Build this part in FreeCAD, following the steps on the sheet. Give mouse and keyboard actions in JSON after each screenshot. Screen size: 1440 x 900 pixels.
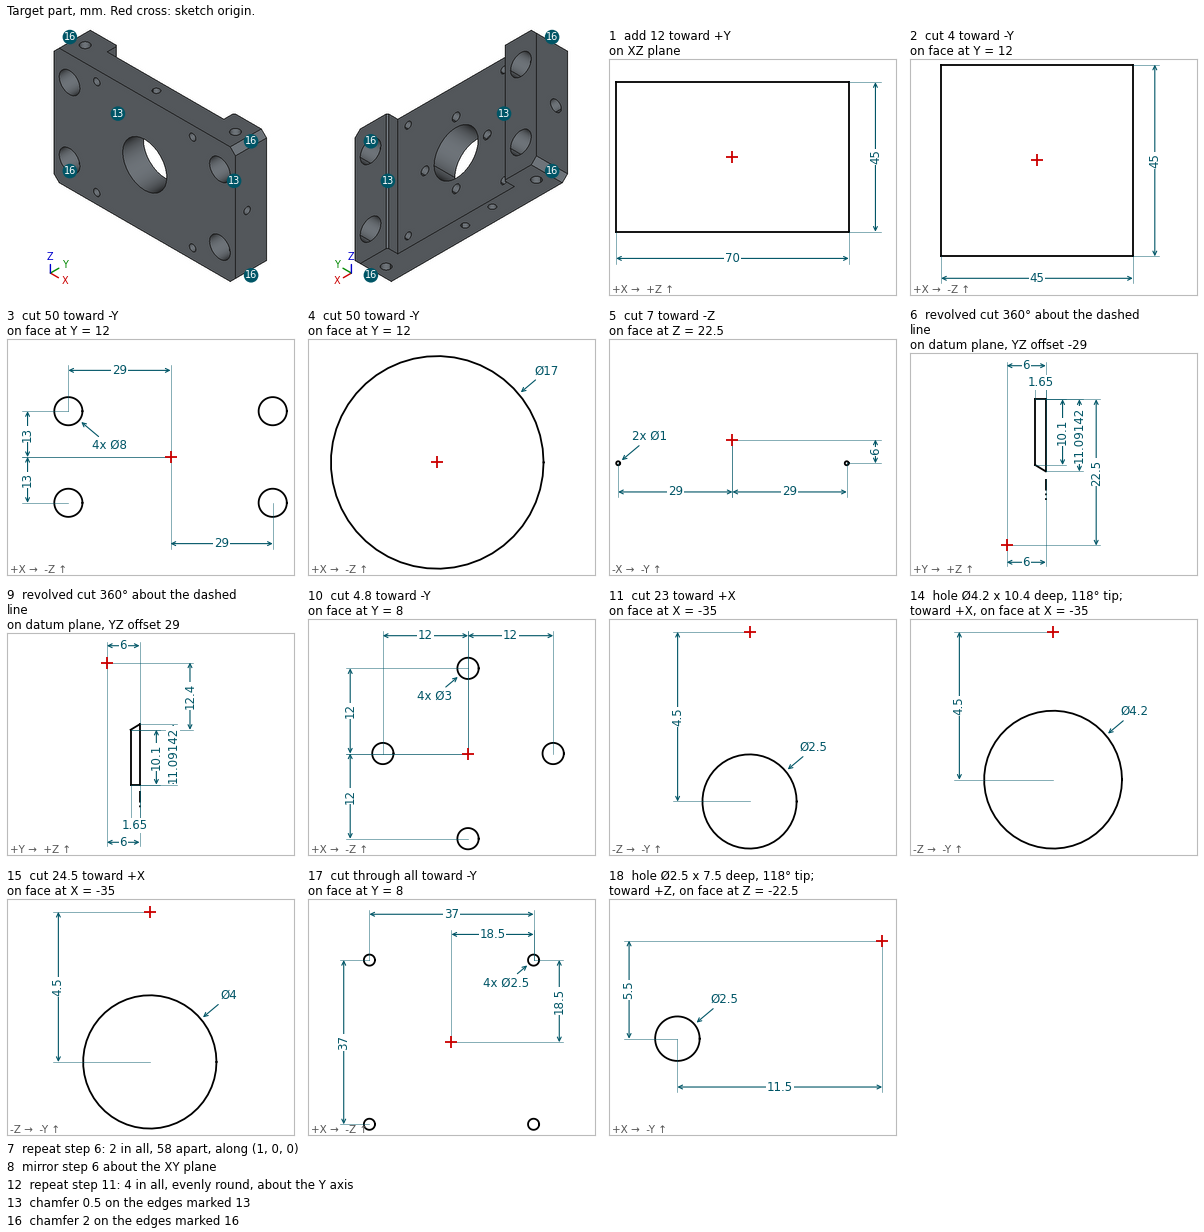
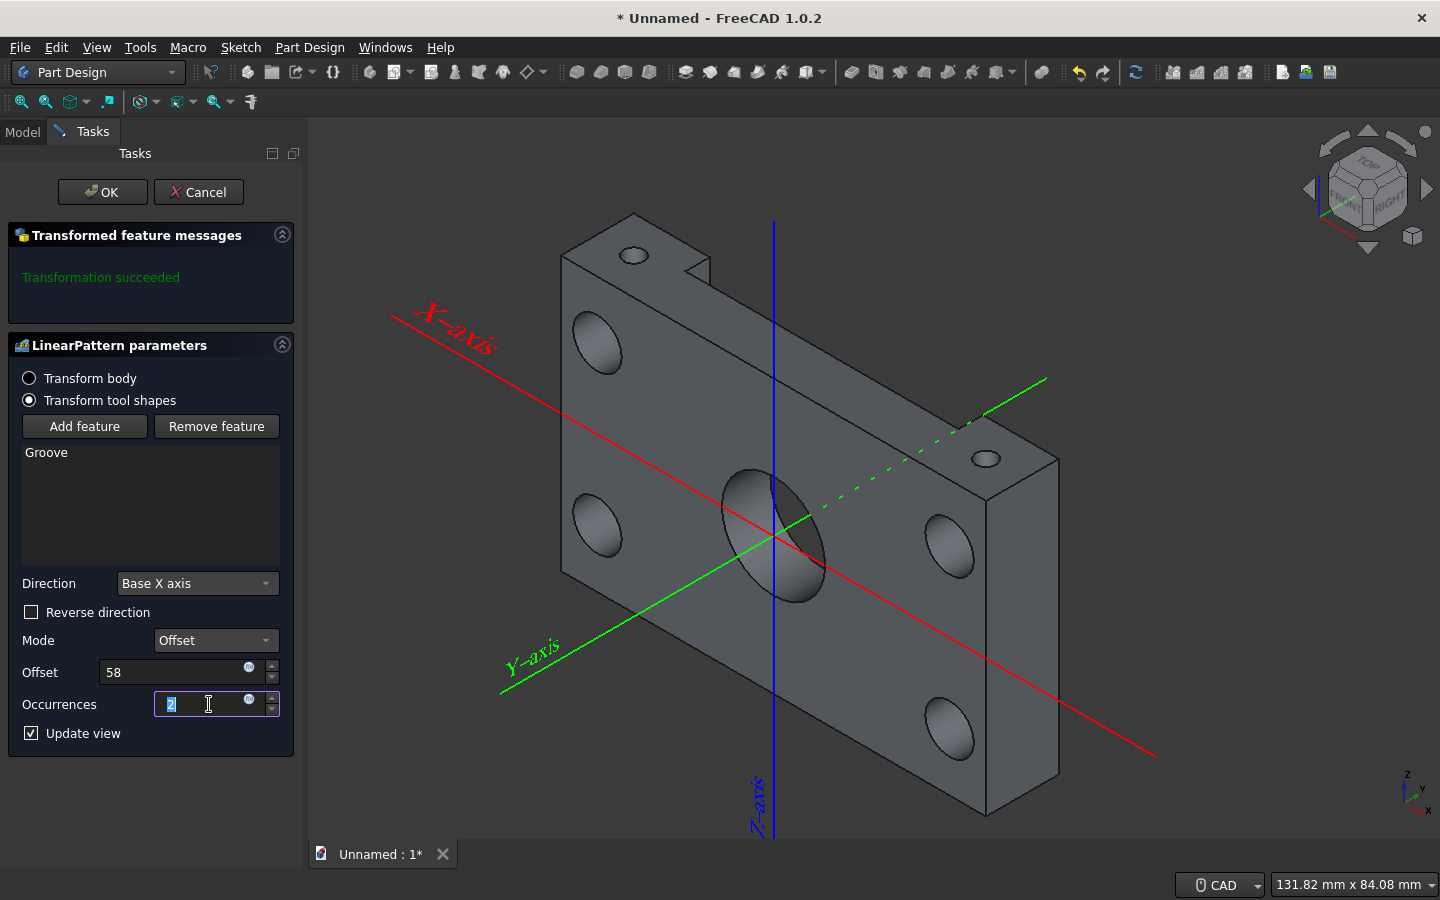
{"action": "type", "text": "2"}
{"action": "key", "text": "Tab"}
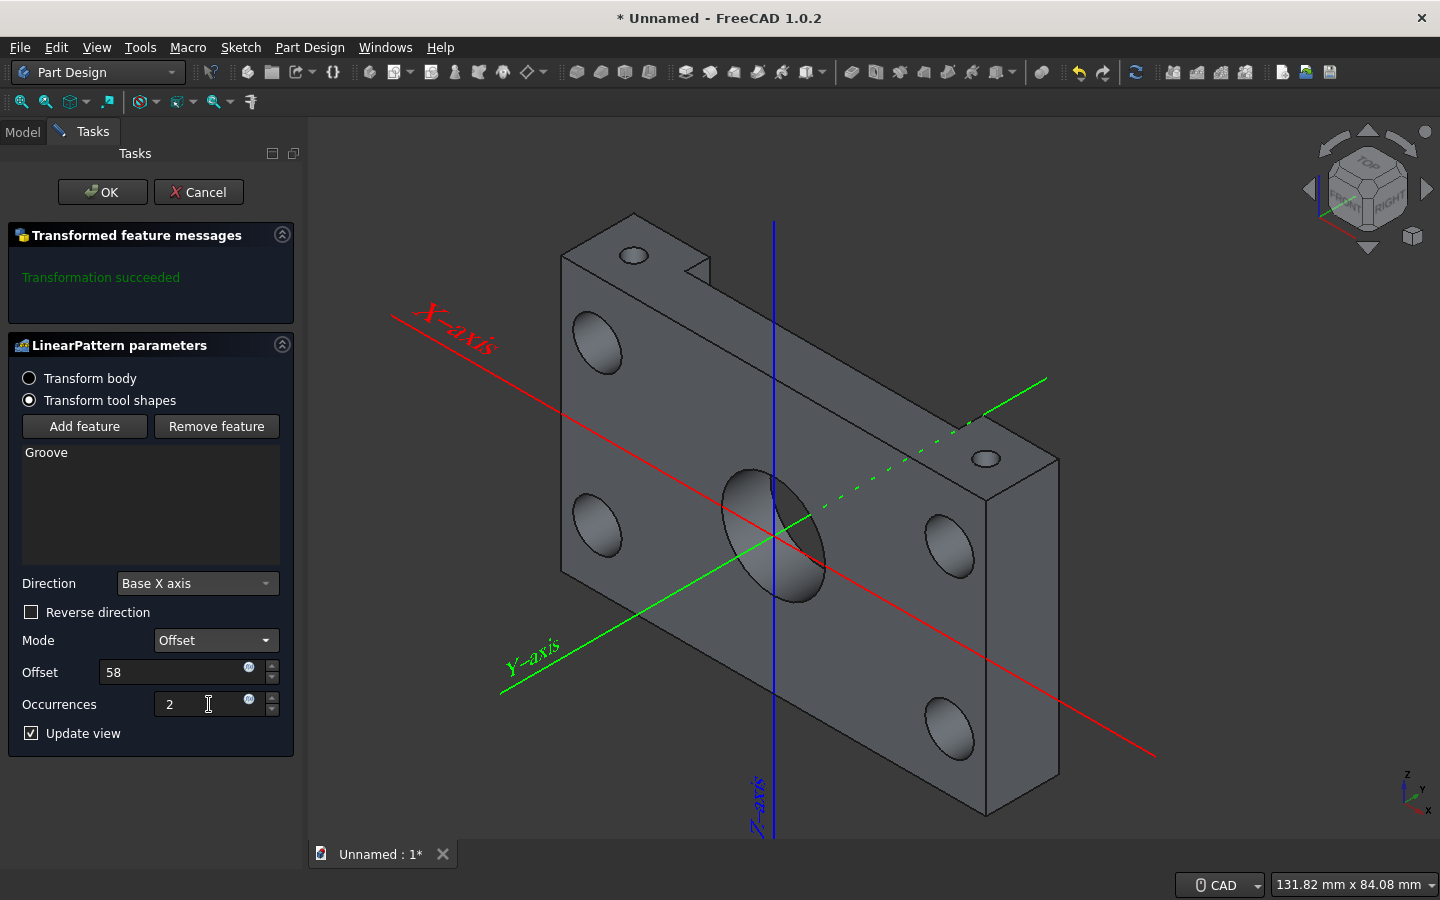
{"action": "left_click", "coordinate": [103, 192]}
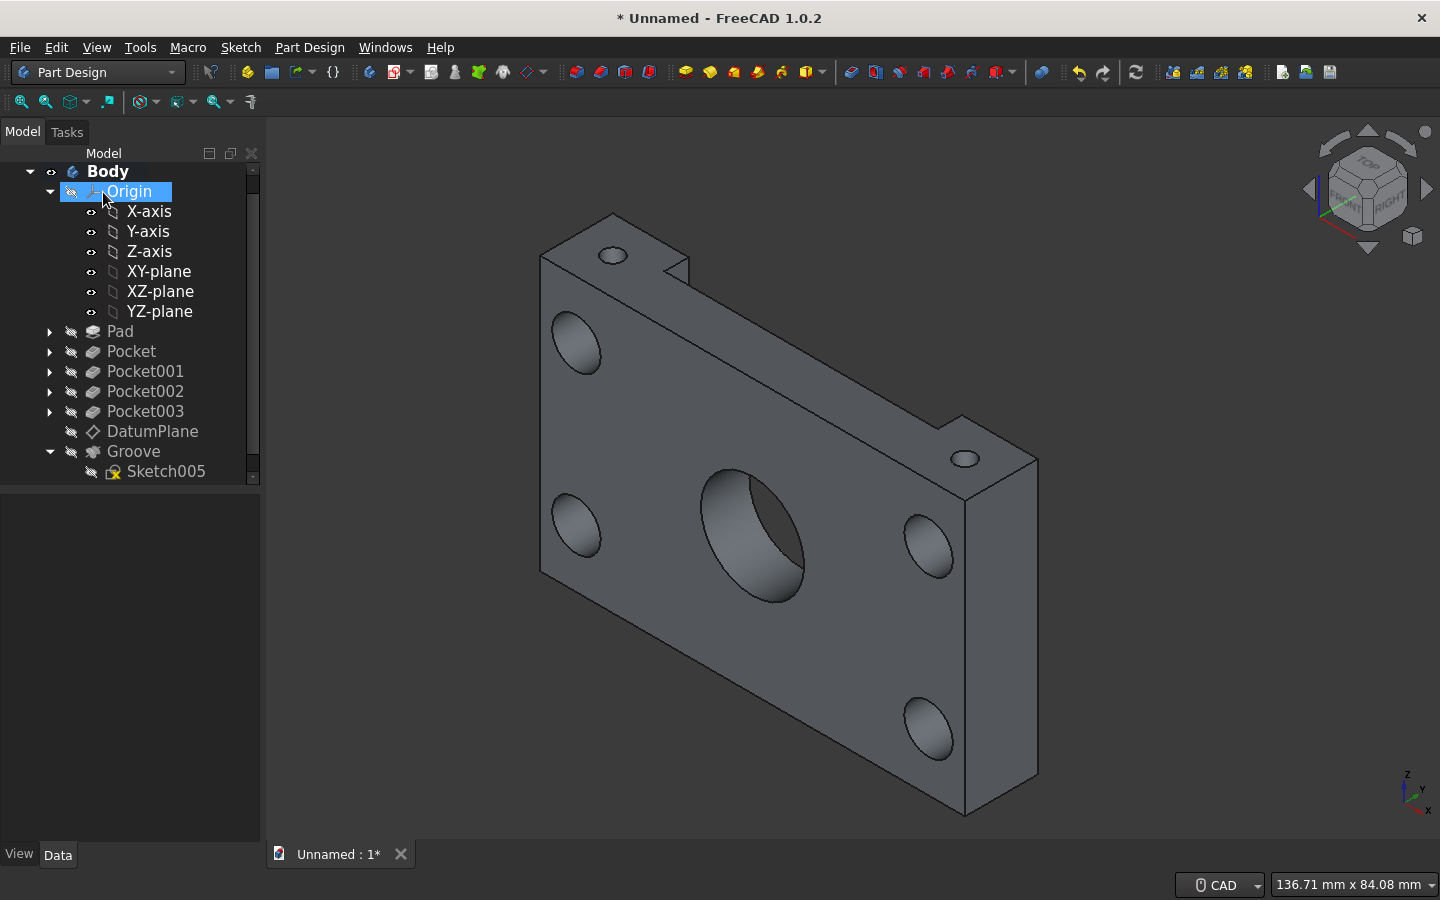
{"action": "left_click", "coordinate": [116, 452]}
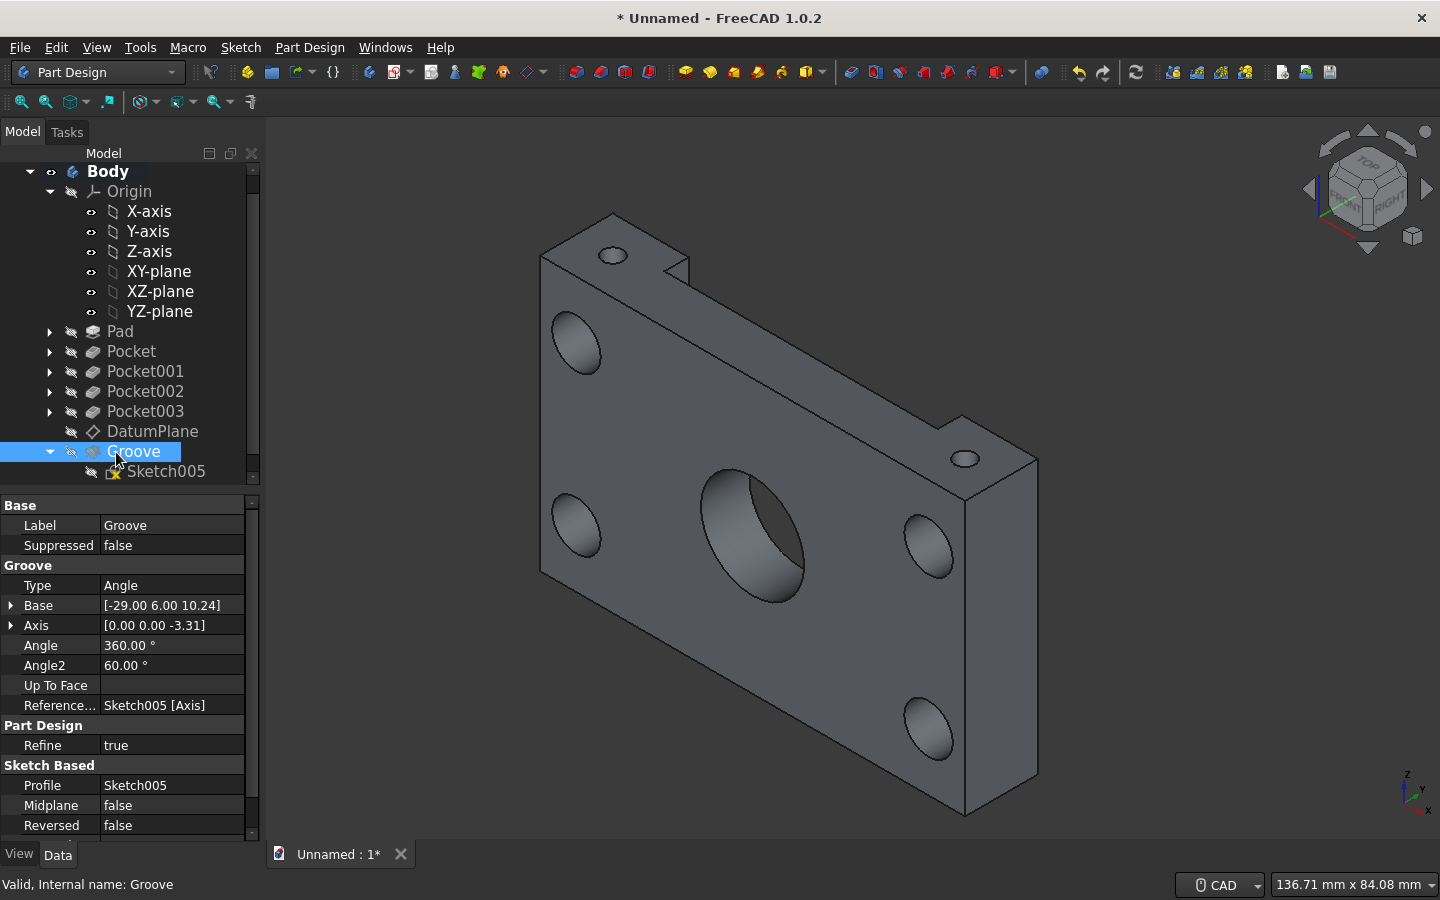
{"action": "left_click", "coordinate": [1174, 72]}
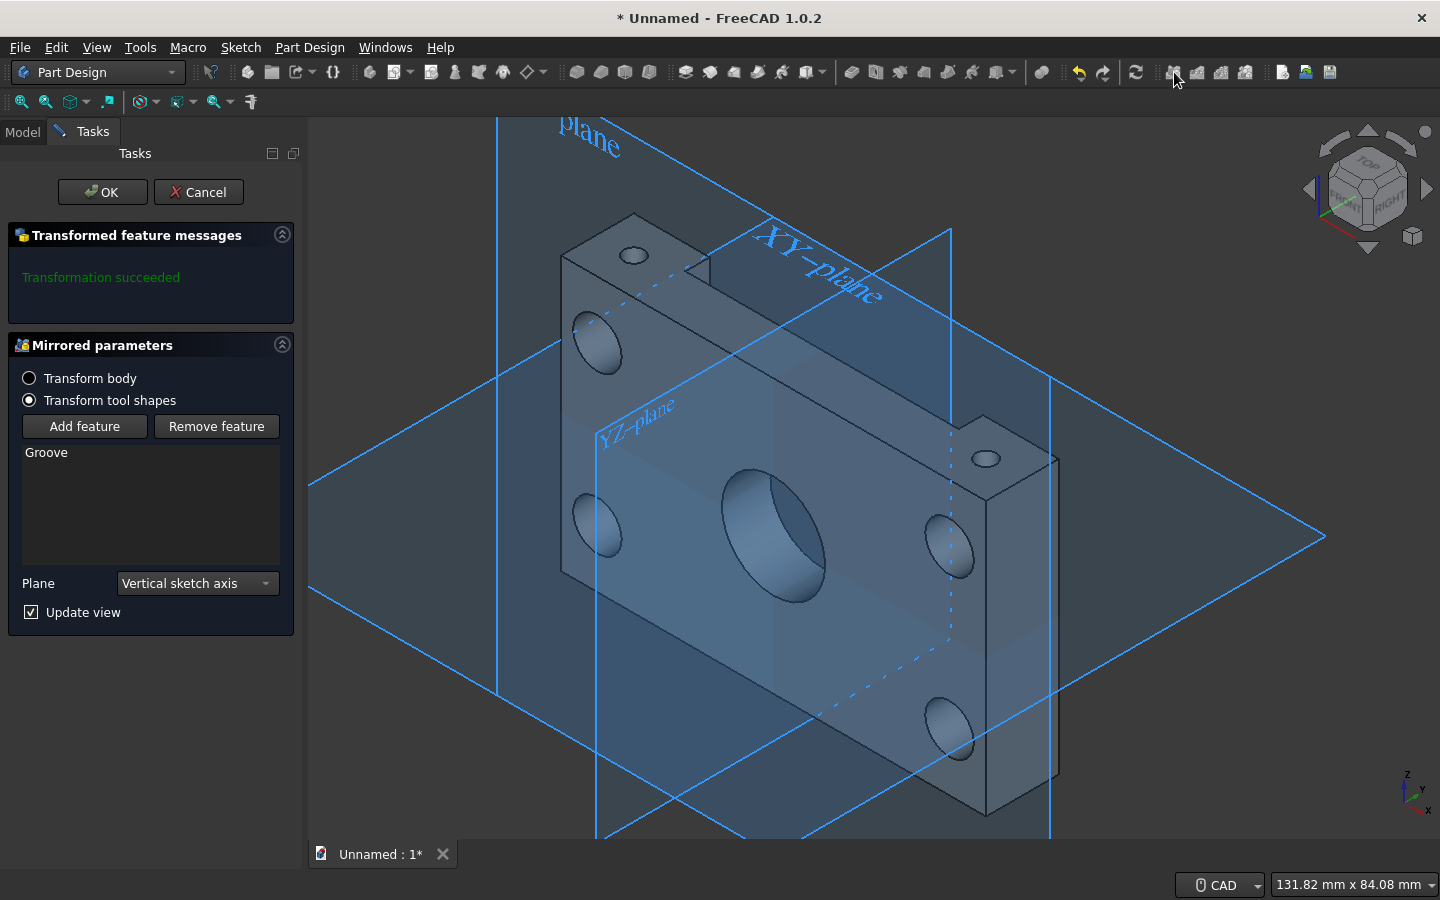
{"action": "left_click", "coordinate": [198, 584]}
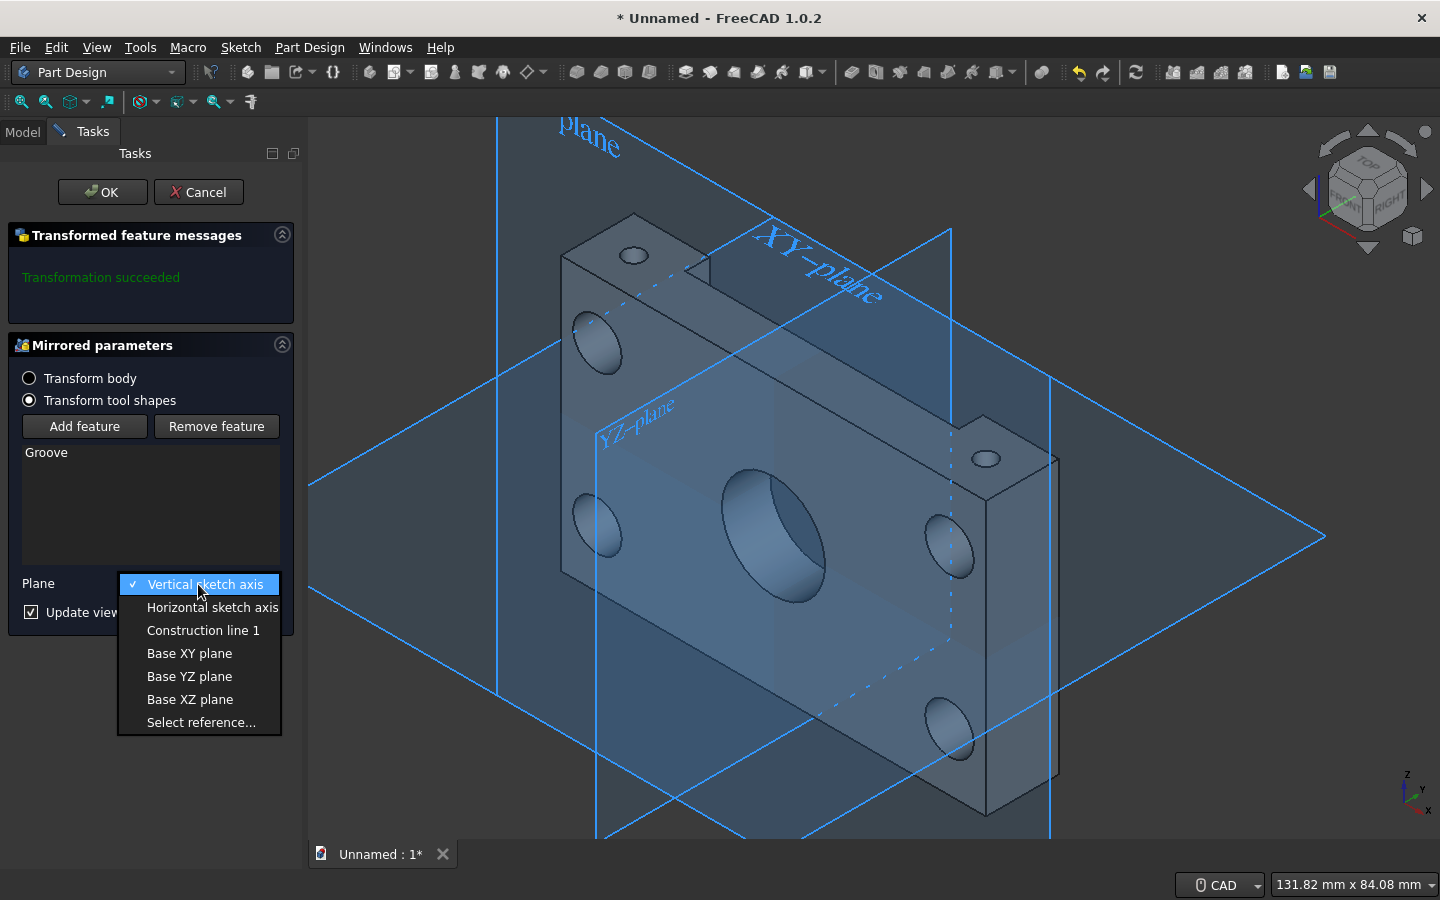
{"action": "left_click", "coordinate": [198, 654]}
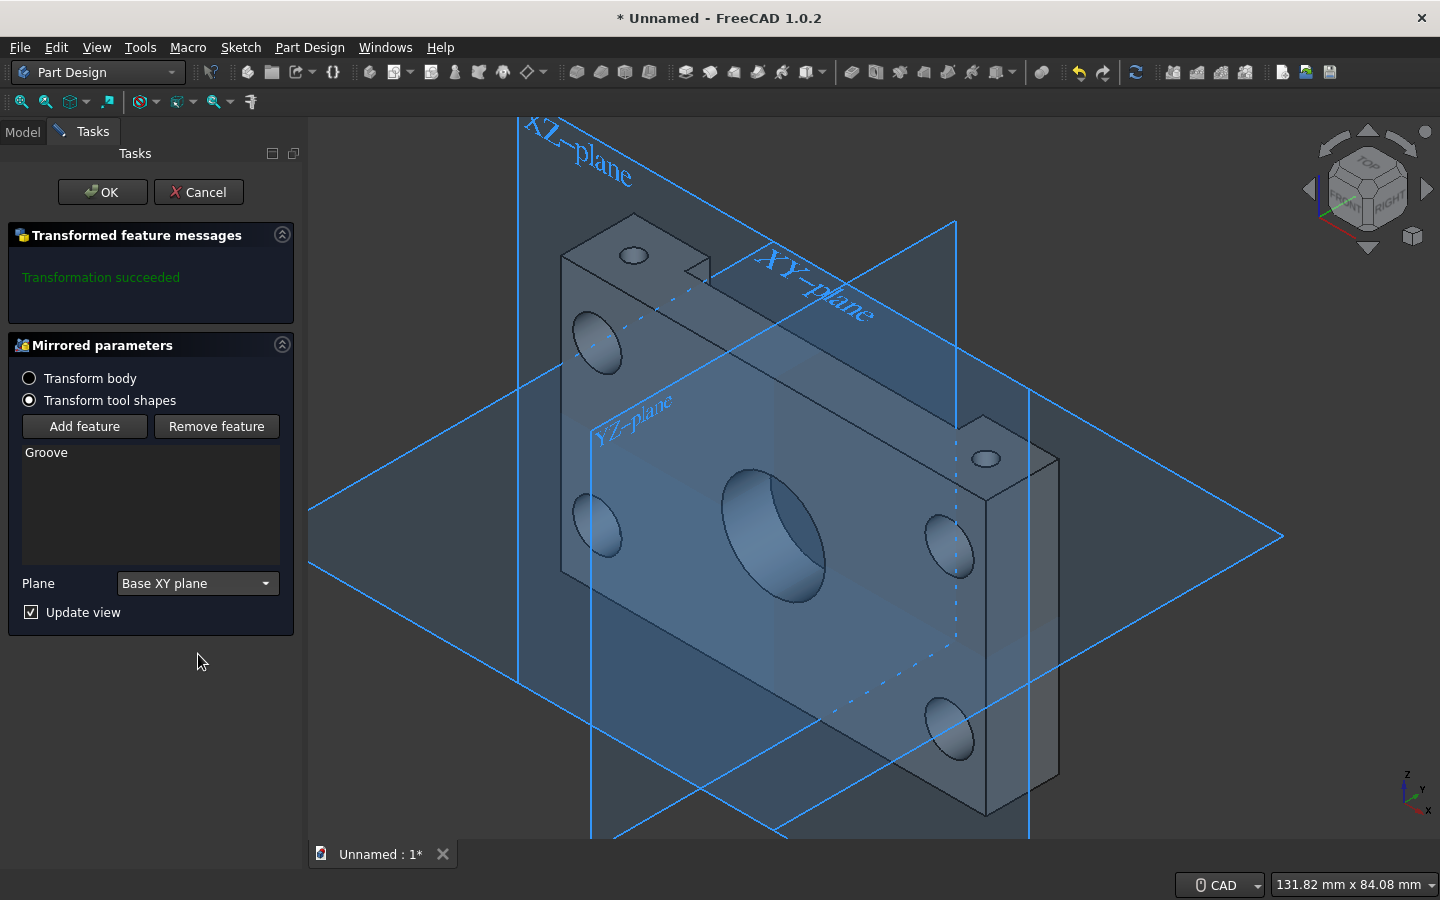
{"action": "left_click", "coordinate": [103, 192]}